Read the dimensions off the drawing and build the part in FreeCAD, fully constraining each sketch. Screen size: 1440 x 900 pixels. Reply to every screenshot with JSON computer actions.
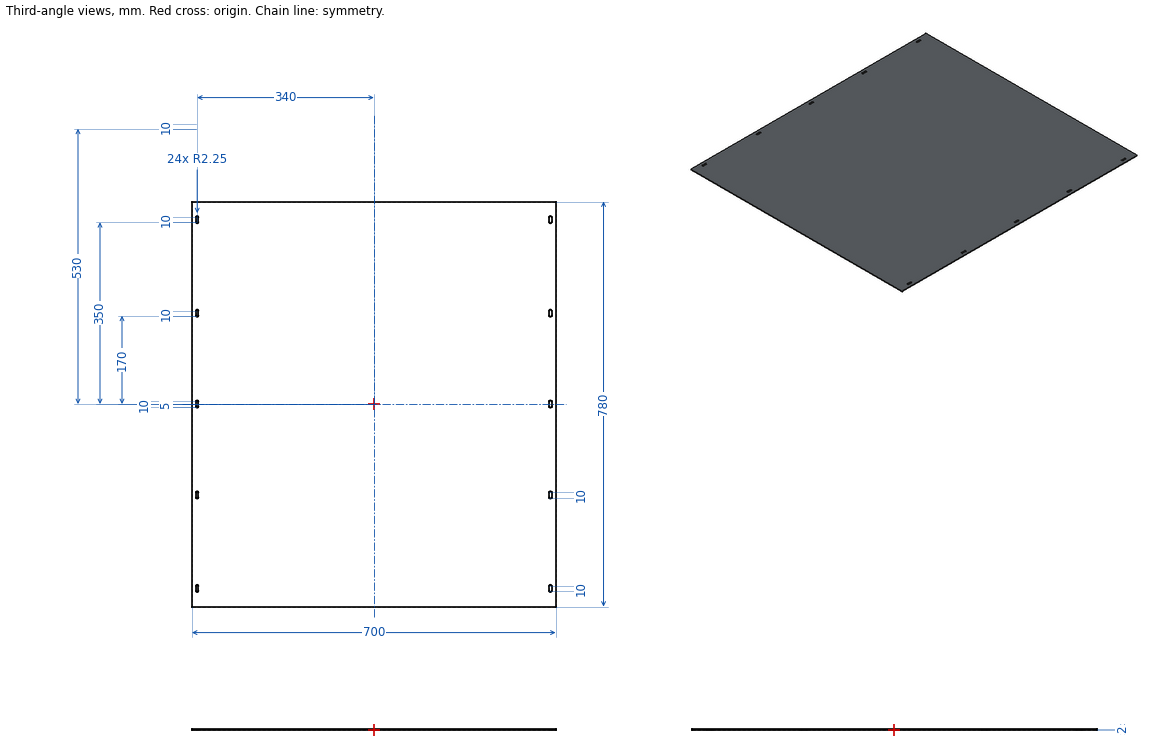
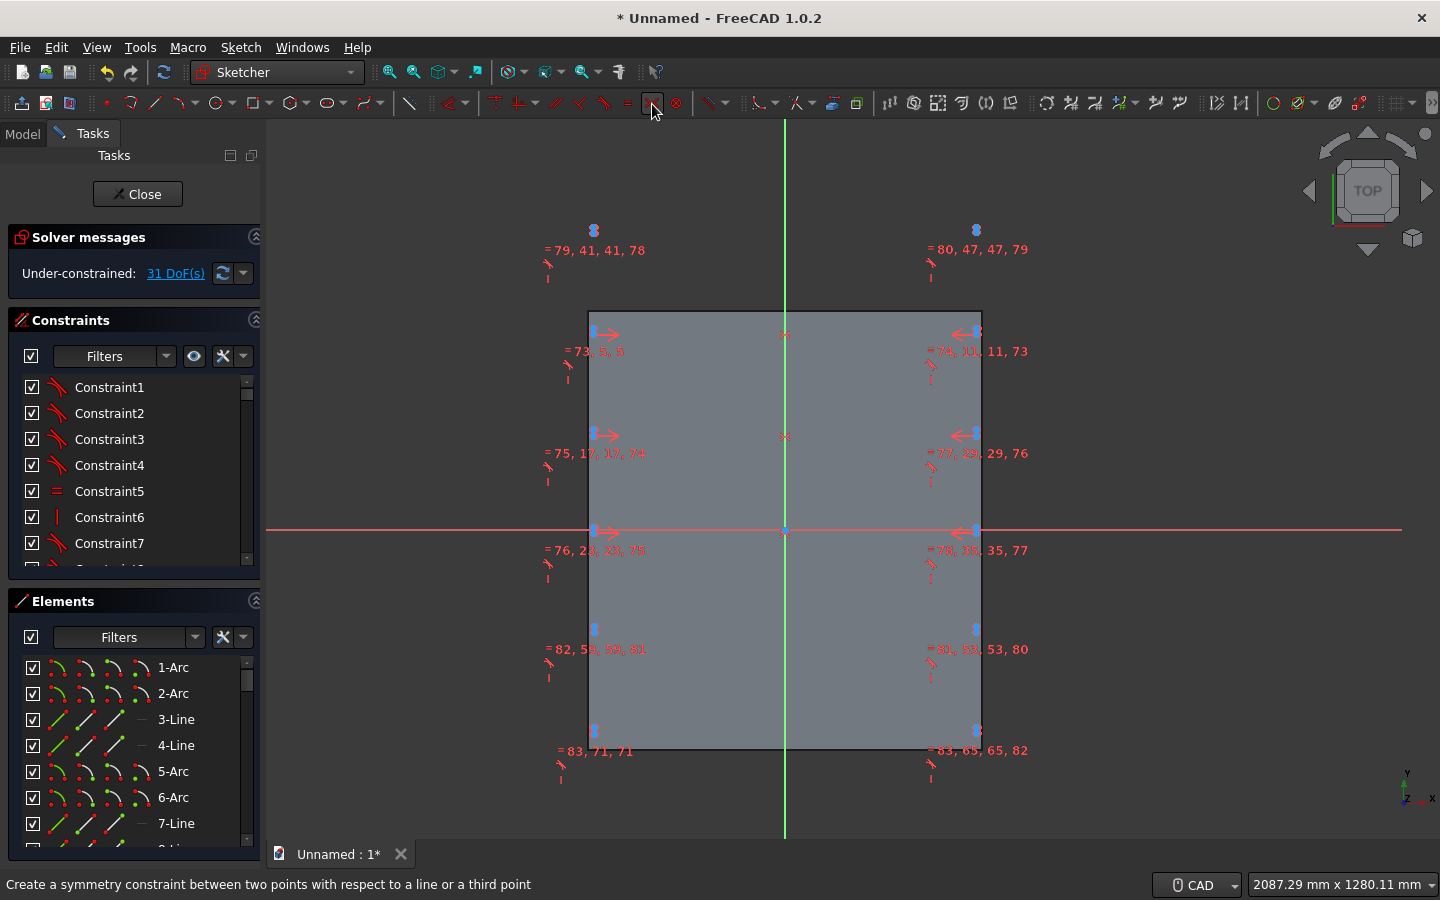
{"action": "scroll", "coordinate": [594, 233], "scroll_direction": "up", "scroll_amount": 12}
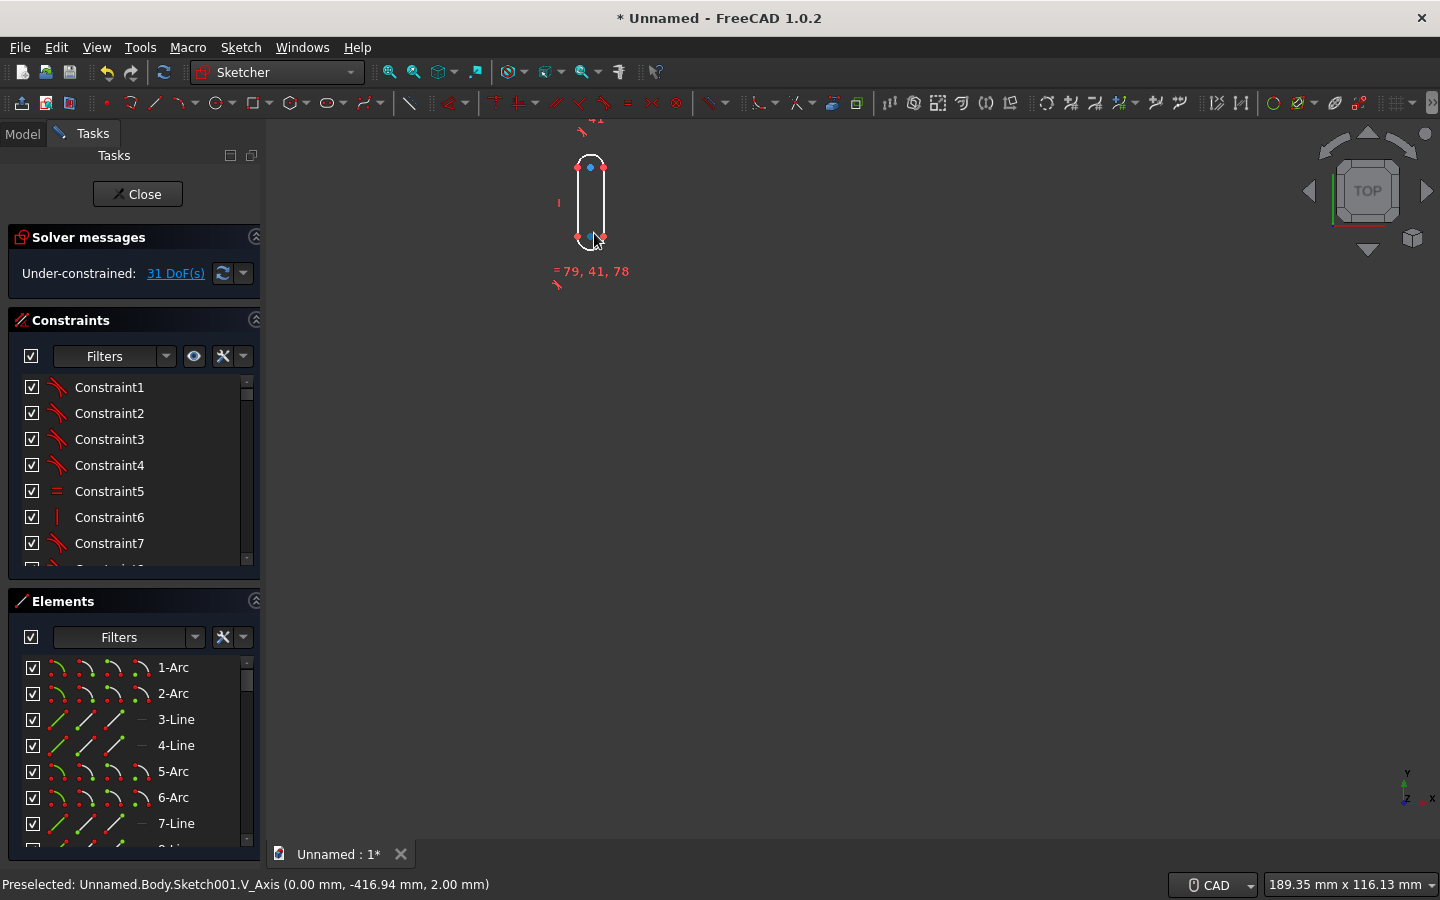
{"action": "left_click", "coordinate": [591, 237]}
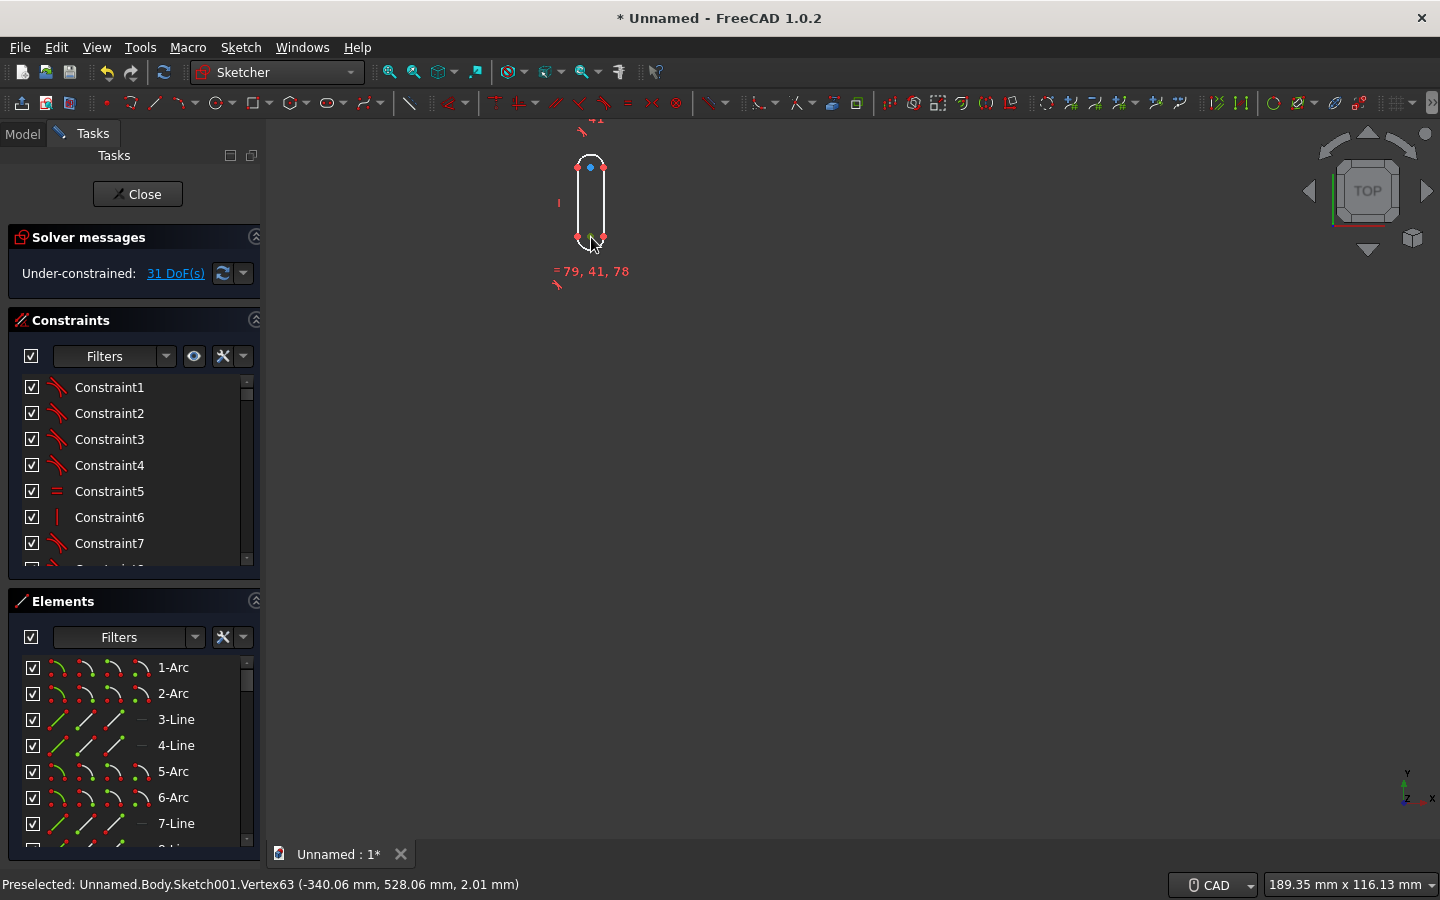
{"action": "scroll", "coordinate": [593, 232], "scroll_direction": "down", "scroll_amount": 12}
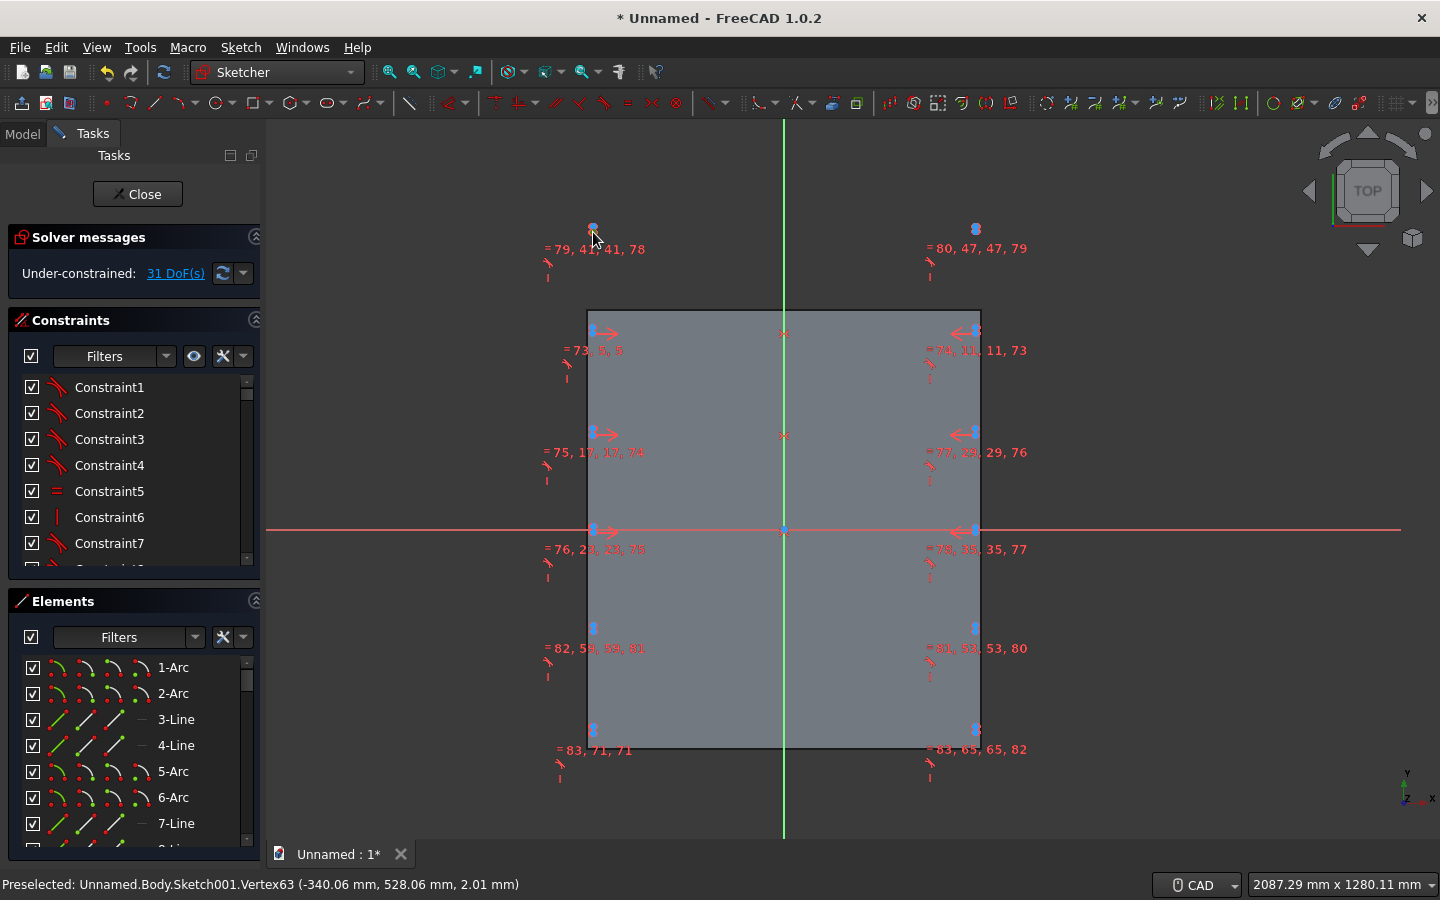
{"action": "scroll", "coordinate": [976, 232], "scroll_direction": "up", "scroll_amount": 12}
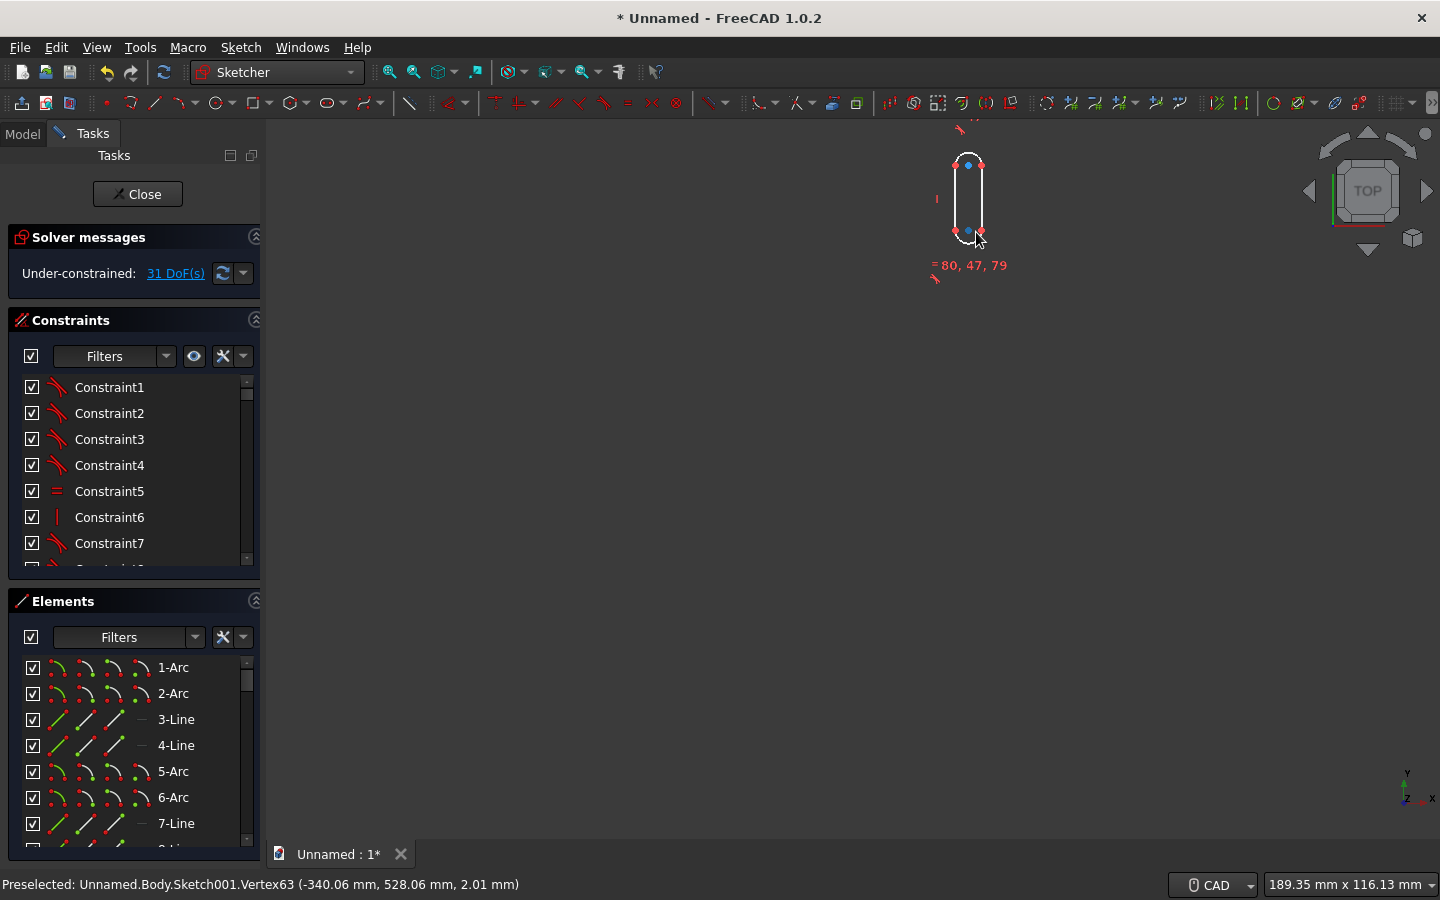
{"action": "left_click", "coordinate": [969, 230]}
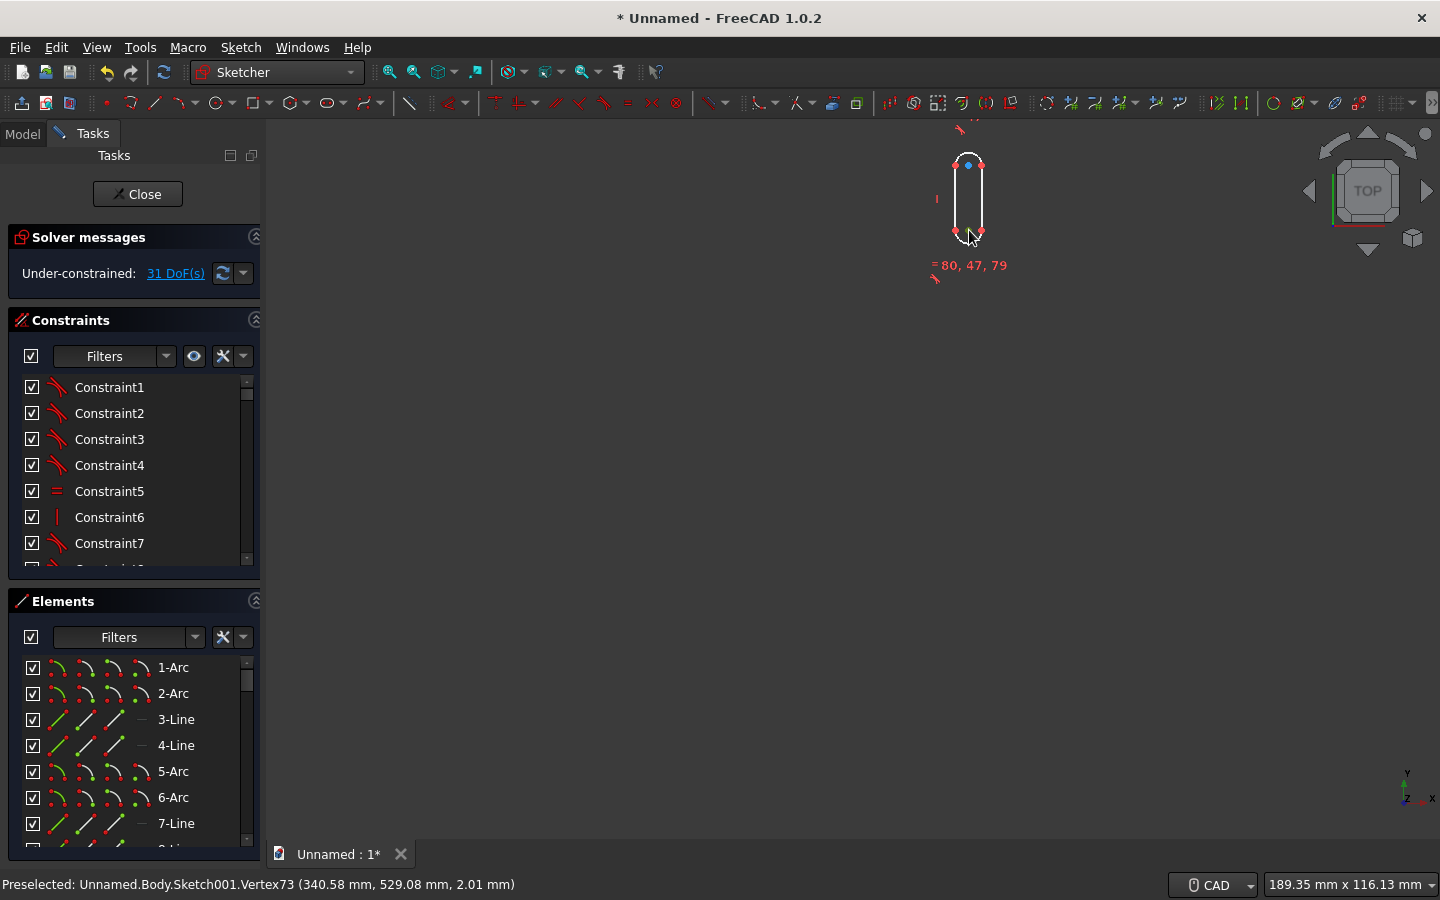
{"action": "scroll", "coordinate": [977, 232], "scroll_direction": "down", "scroll_amount": 12}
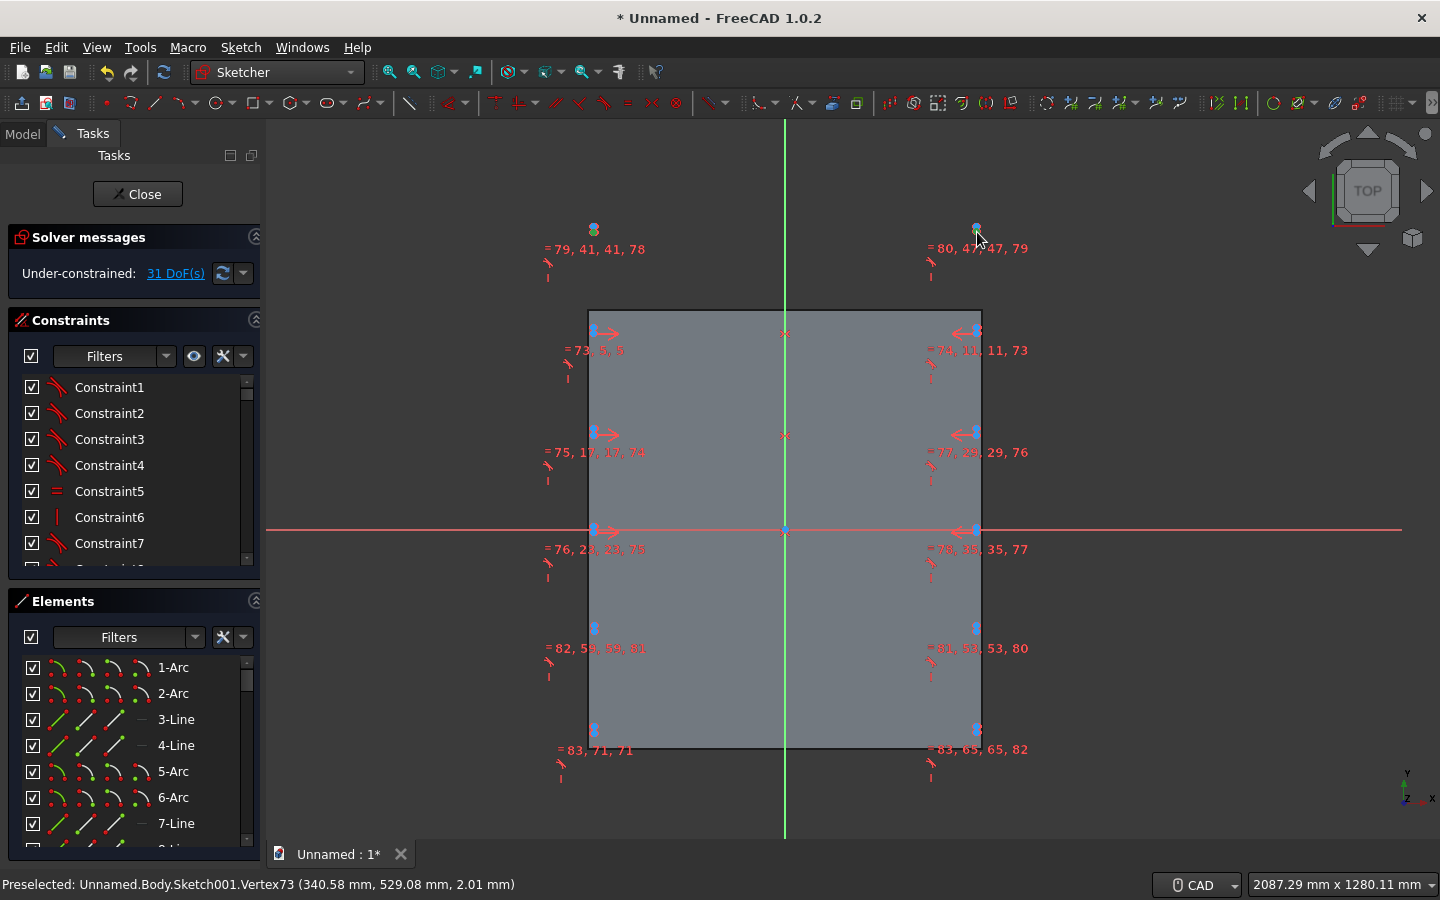
{"action": "left_click", "coordinate": [785, 764]}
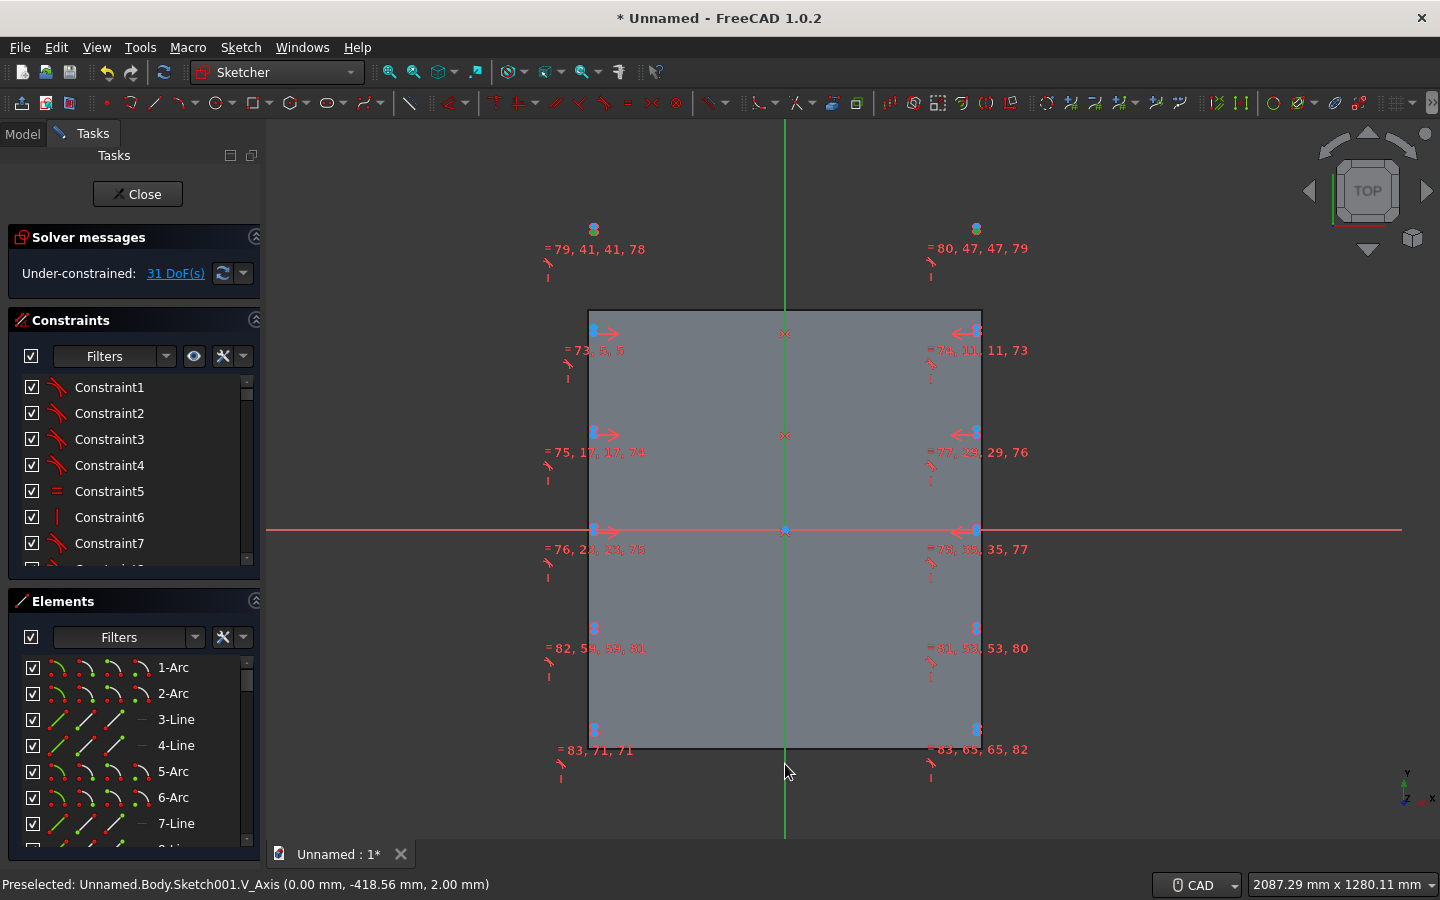
{"action": "key", "text": "s"}